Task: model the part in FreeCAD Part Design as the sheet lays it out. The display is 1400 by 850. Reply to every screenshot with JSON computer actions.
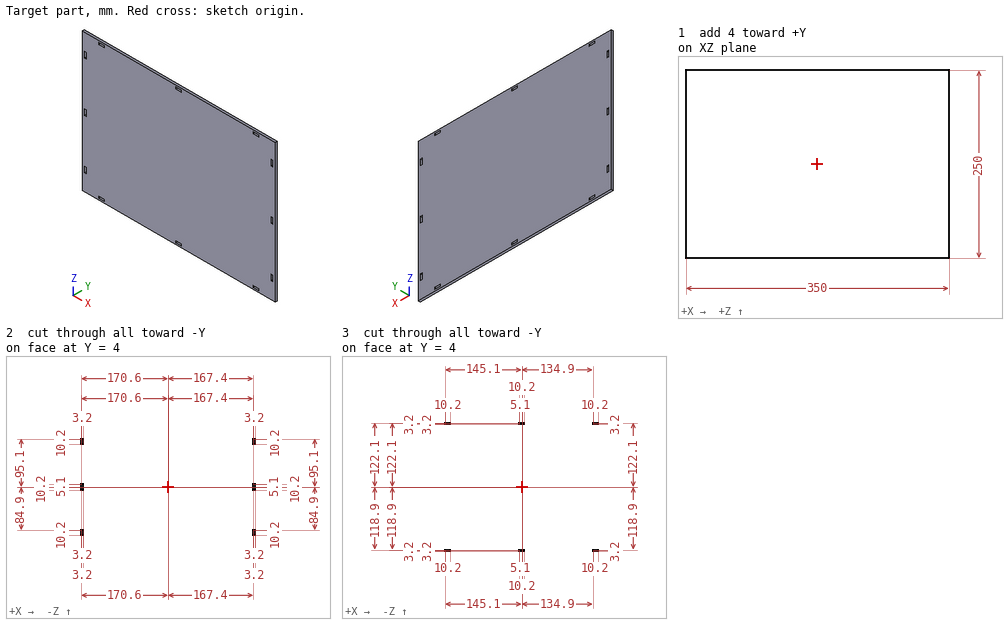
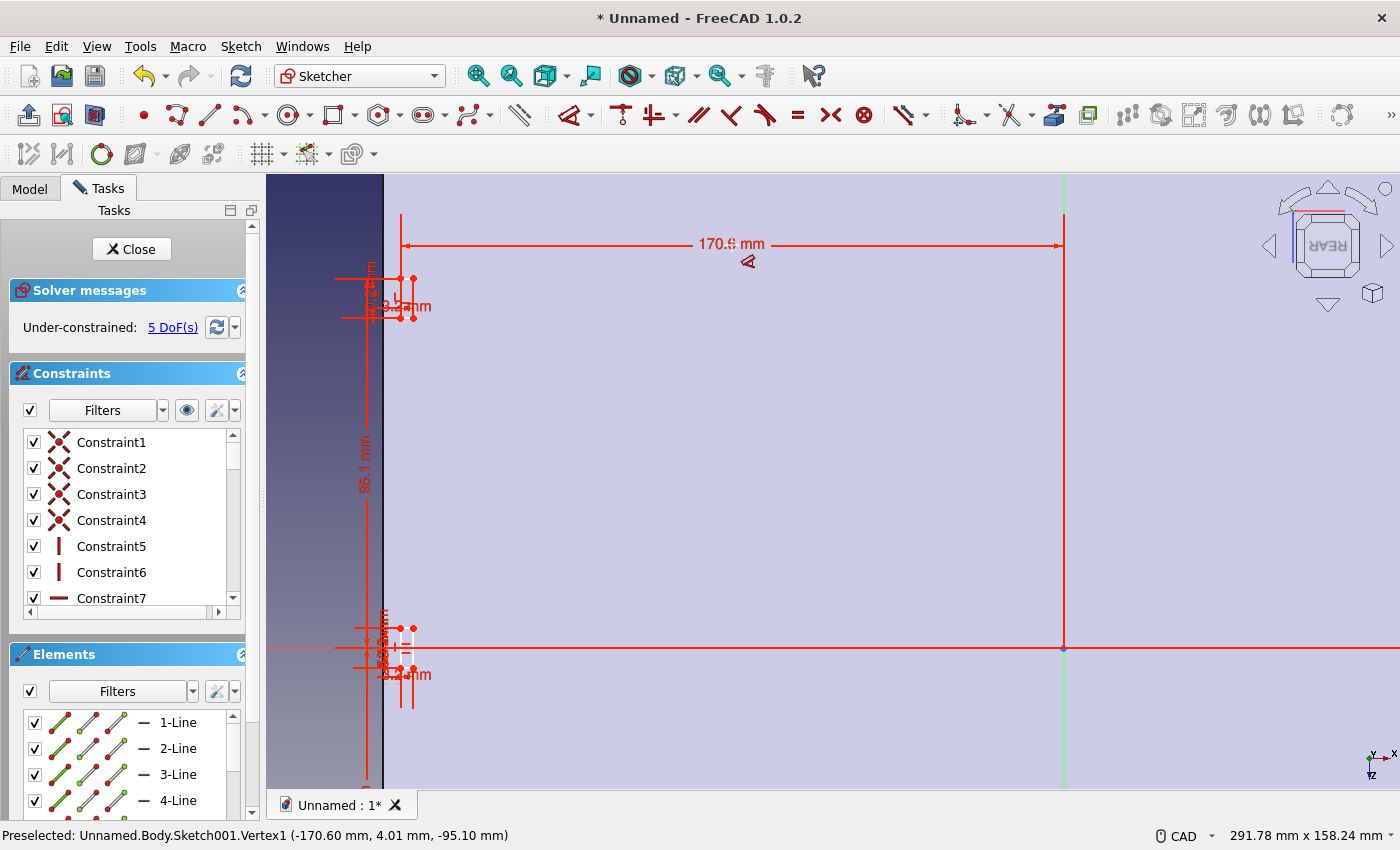
{"action": "left_click", "coordinate": [401, 628]}
{"action": "left_click", "coordinate": [732, 594]}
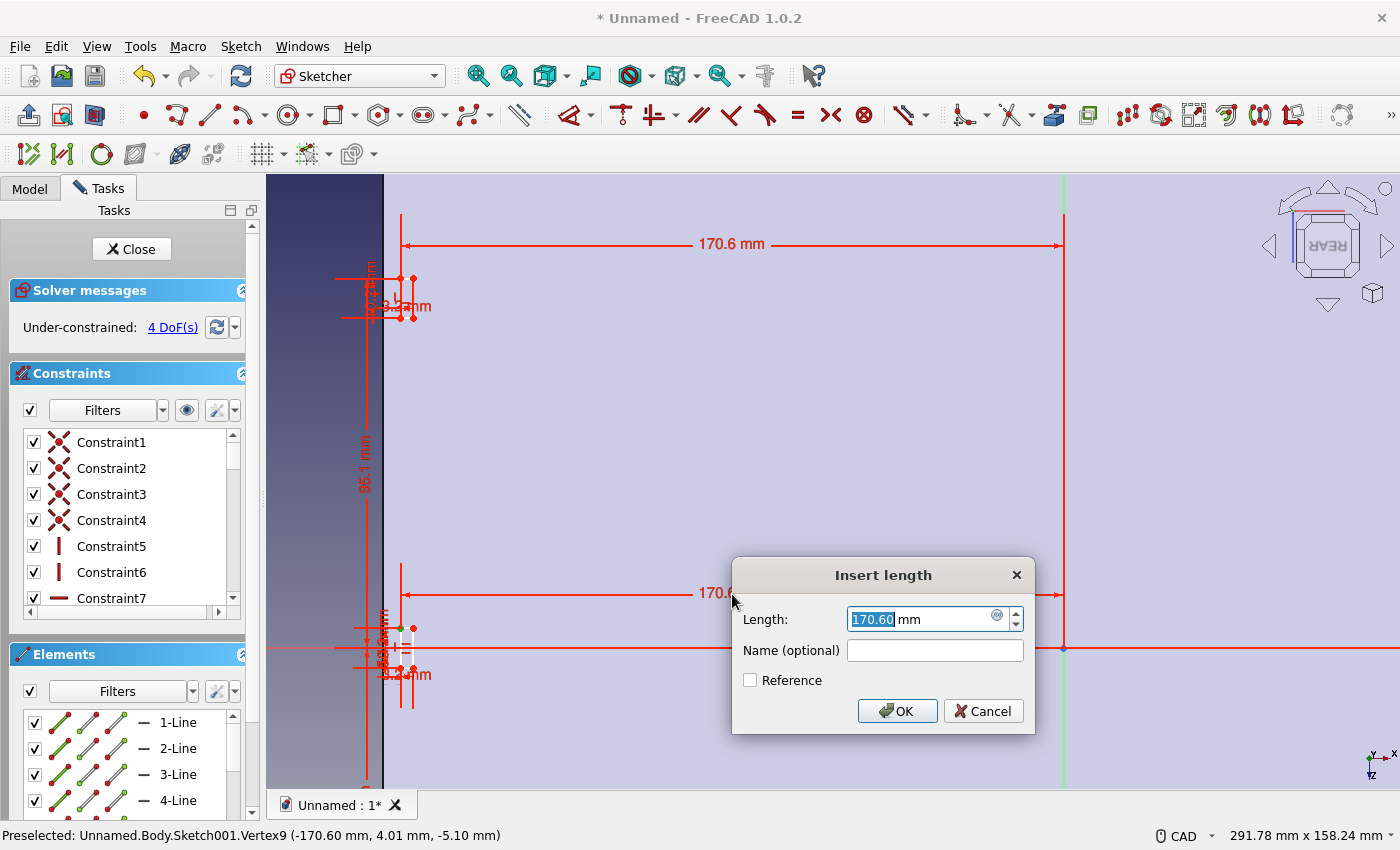
{"action": "type", "text": "170.6"}
{"action": "key", "text": "Return"}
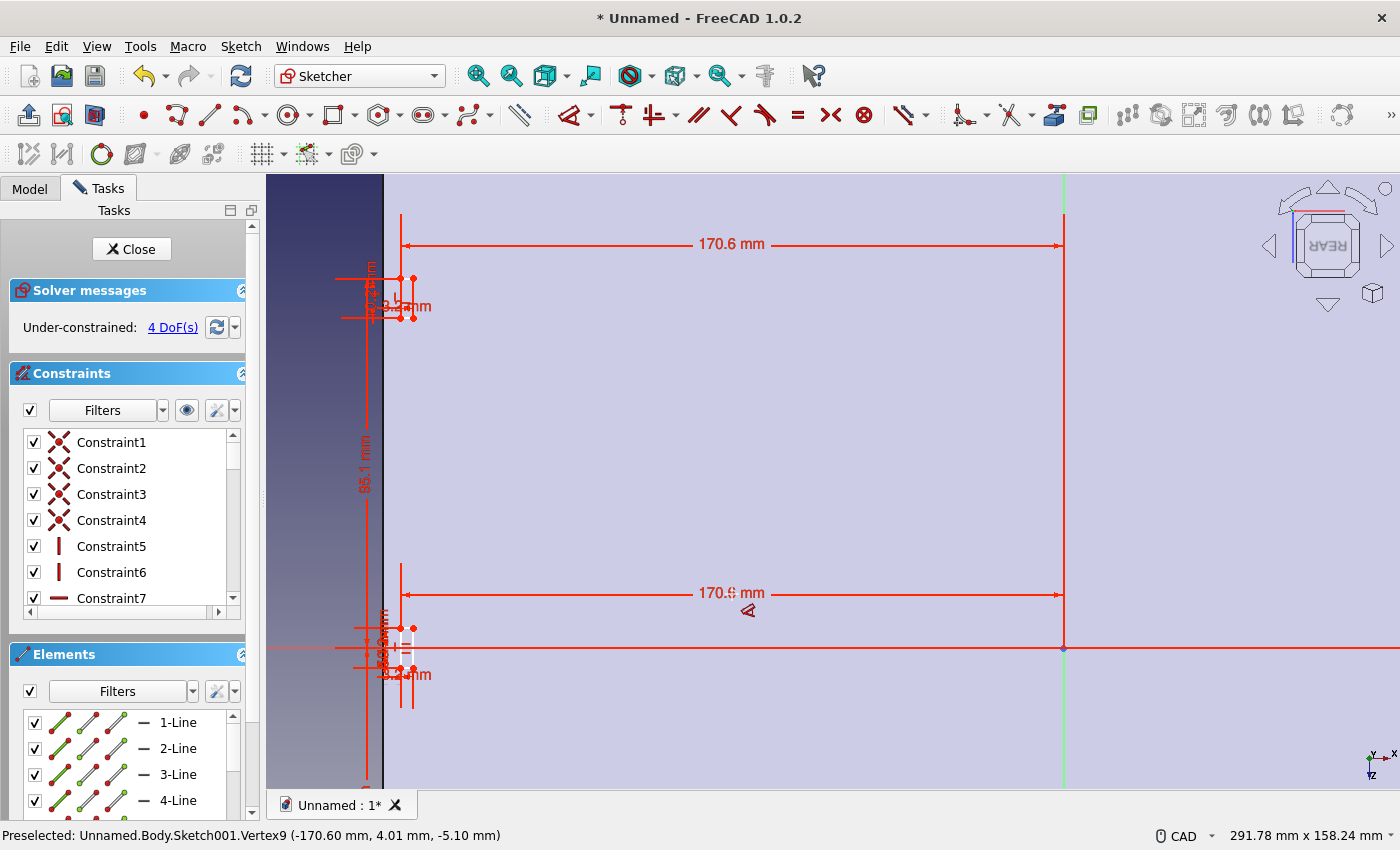
{"action": "scroll", "coordinate": [401, 279], "scroll_direction": "down", "scroll_amount": 3}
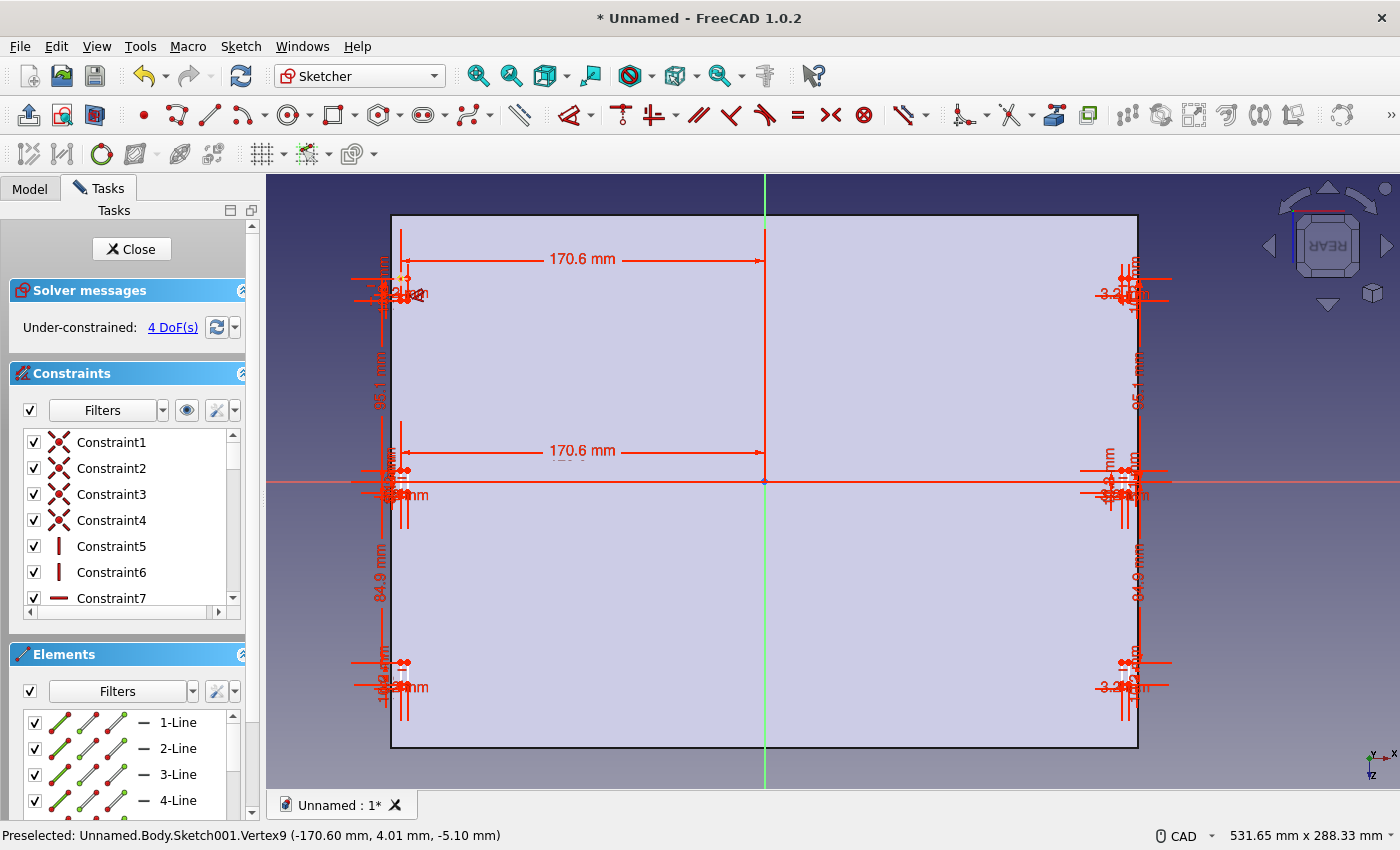
{"action": "scroll", "coordinate": [401, 663], "scroll_direction": "up", "scroll_amount": 3}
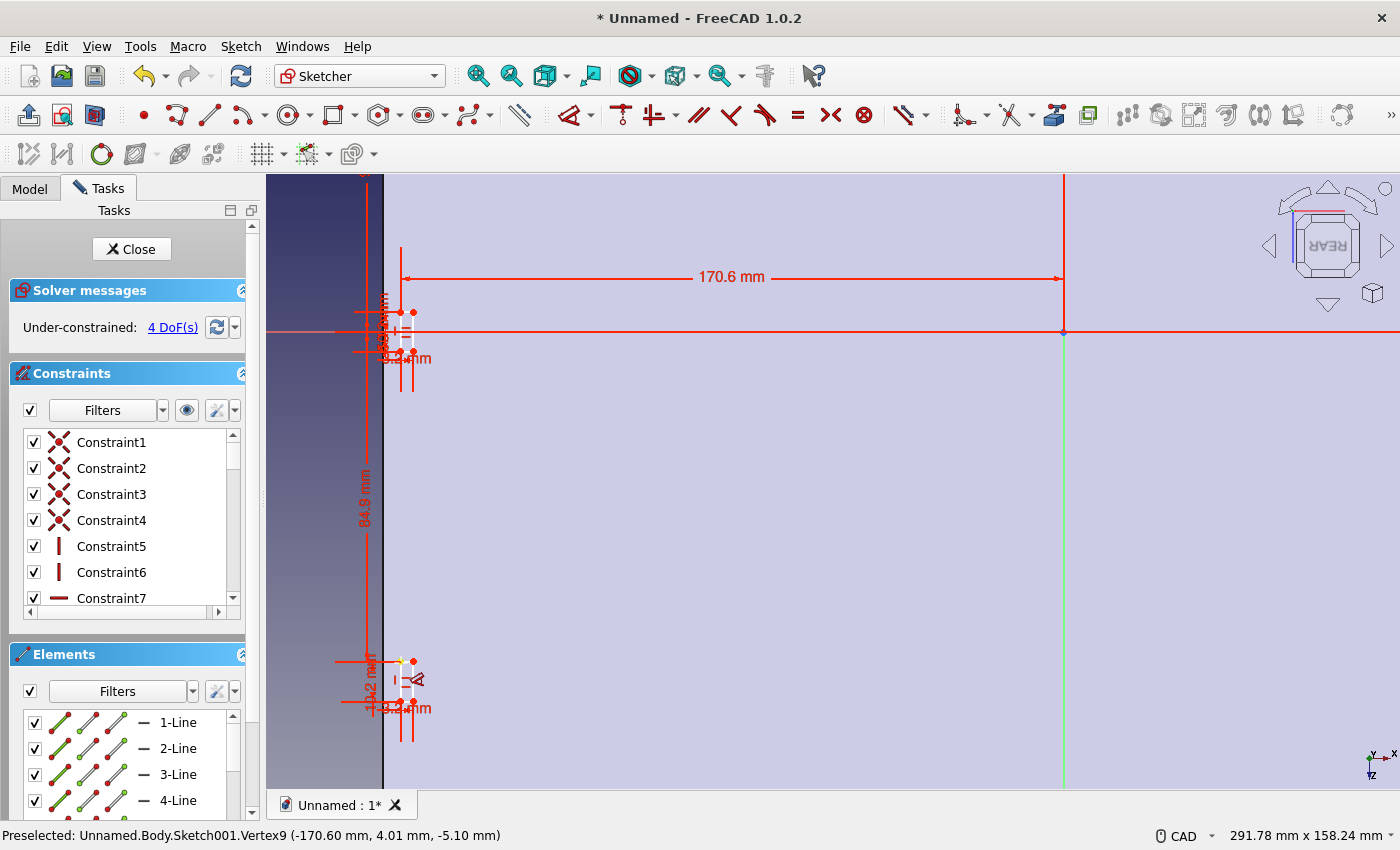
{"action": "left_click", "coordinate": [401, 662]}
{"action": "left_click", "coordinate": [732, 696]}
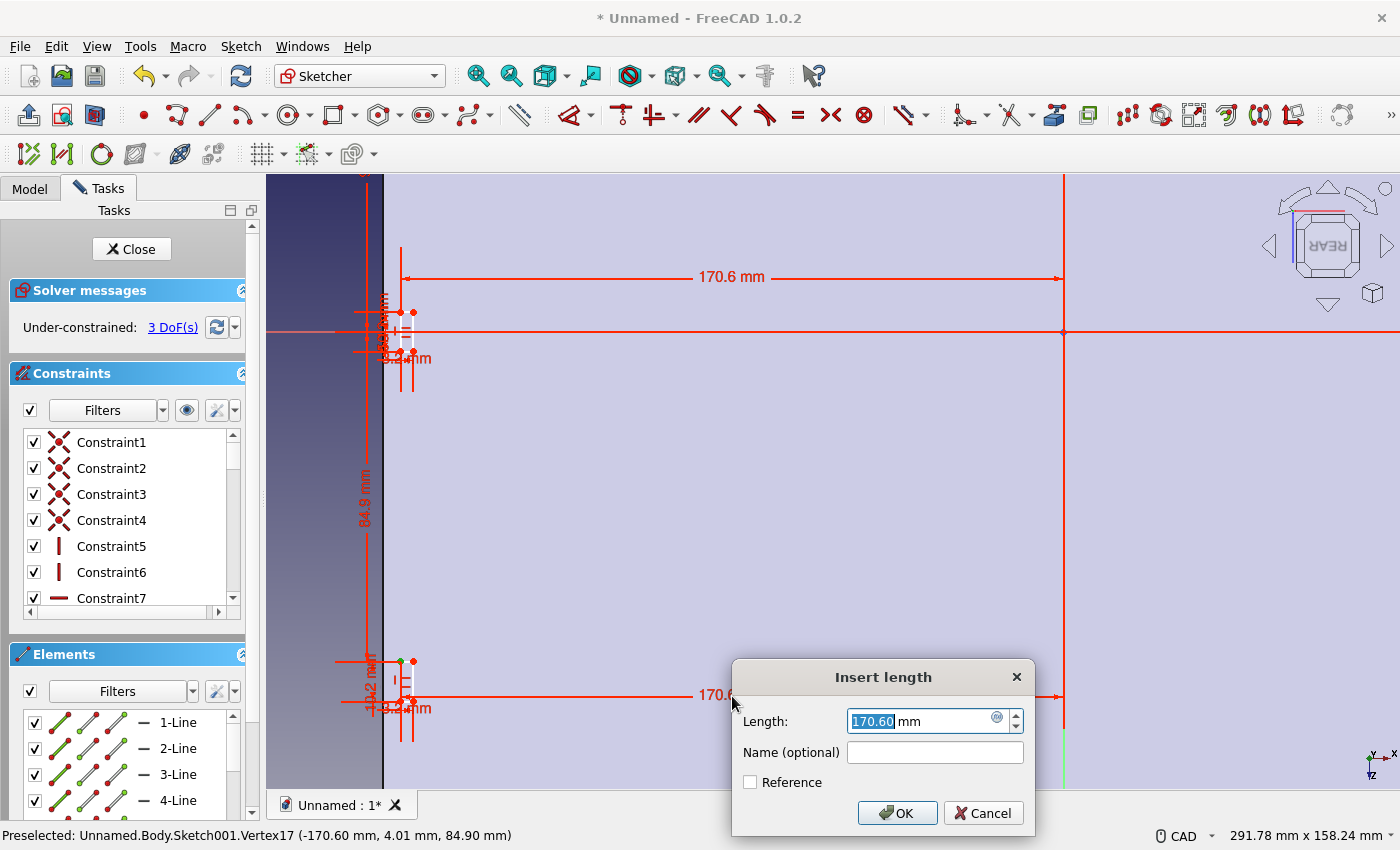
{"action": "type", "text": "170.6"}
{"action": "key", "text": "Return"}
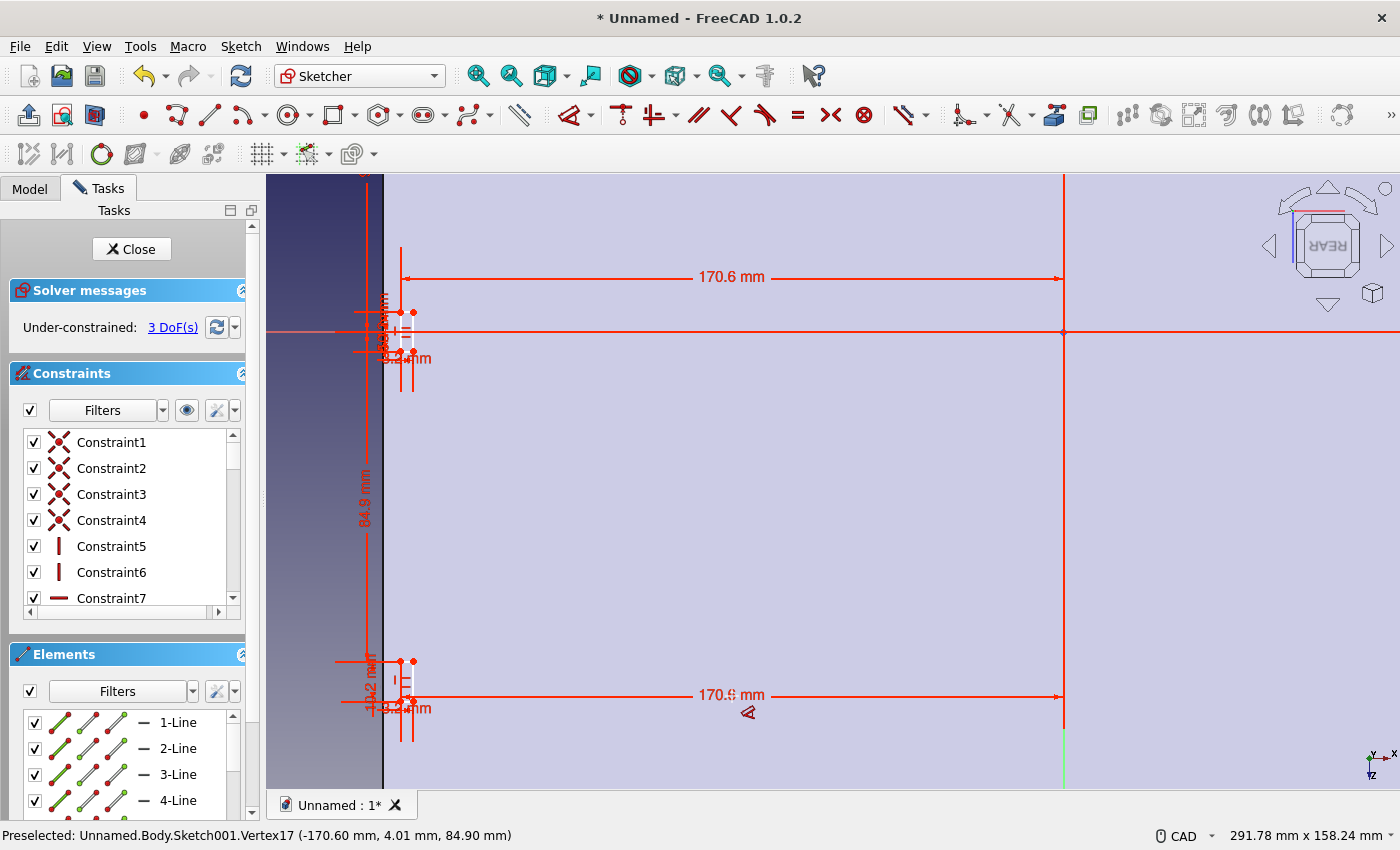
{"action": "scroll", "coordinate": [401, 663], "scroll_direction": "down", "scroll_amount": 3}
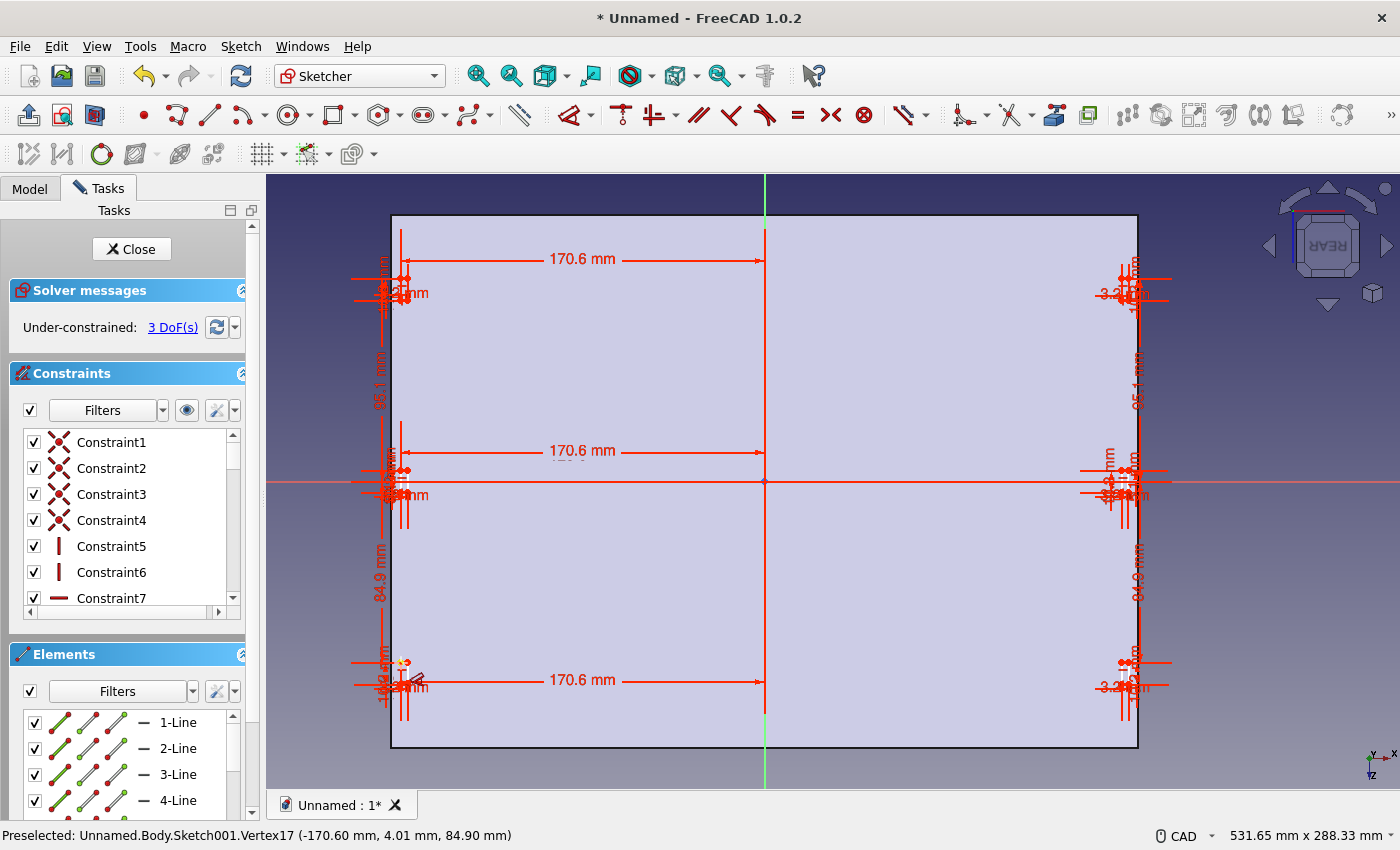
{"action": "scroll", "coordinate": [1122, 663], "scroll_direction": "up", "scroll_amount": 3}